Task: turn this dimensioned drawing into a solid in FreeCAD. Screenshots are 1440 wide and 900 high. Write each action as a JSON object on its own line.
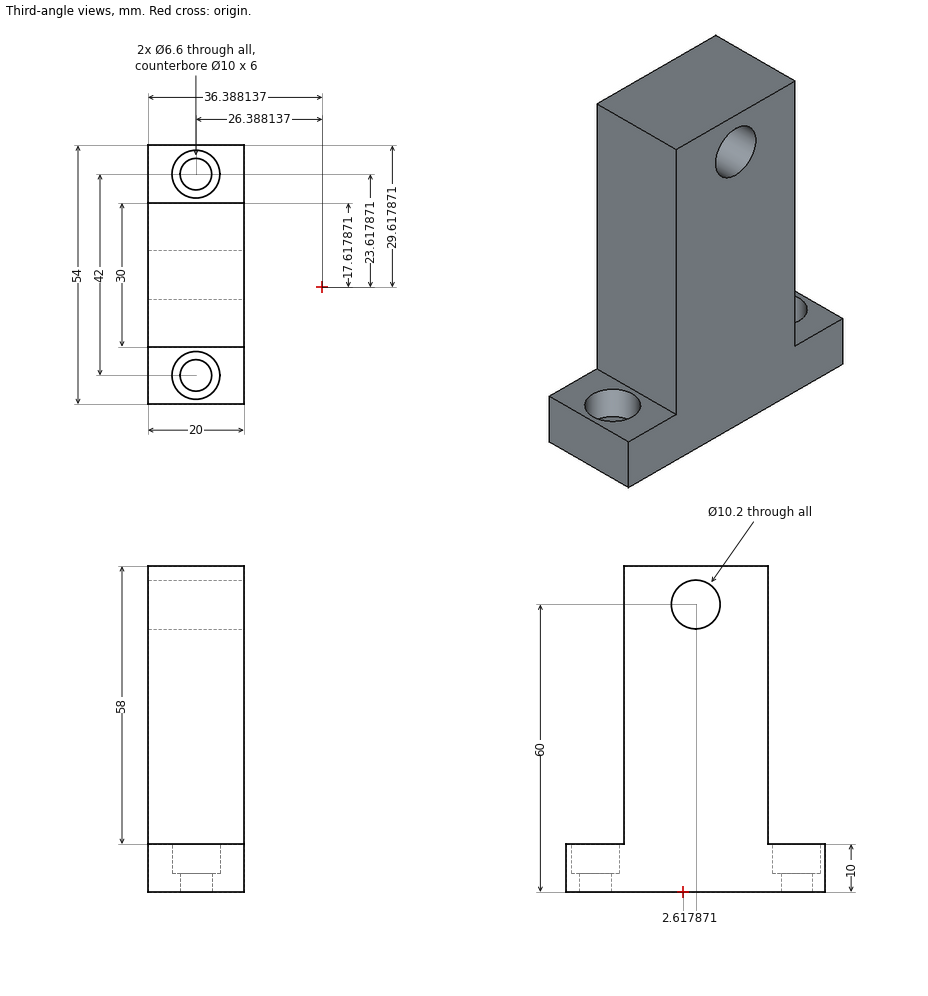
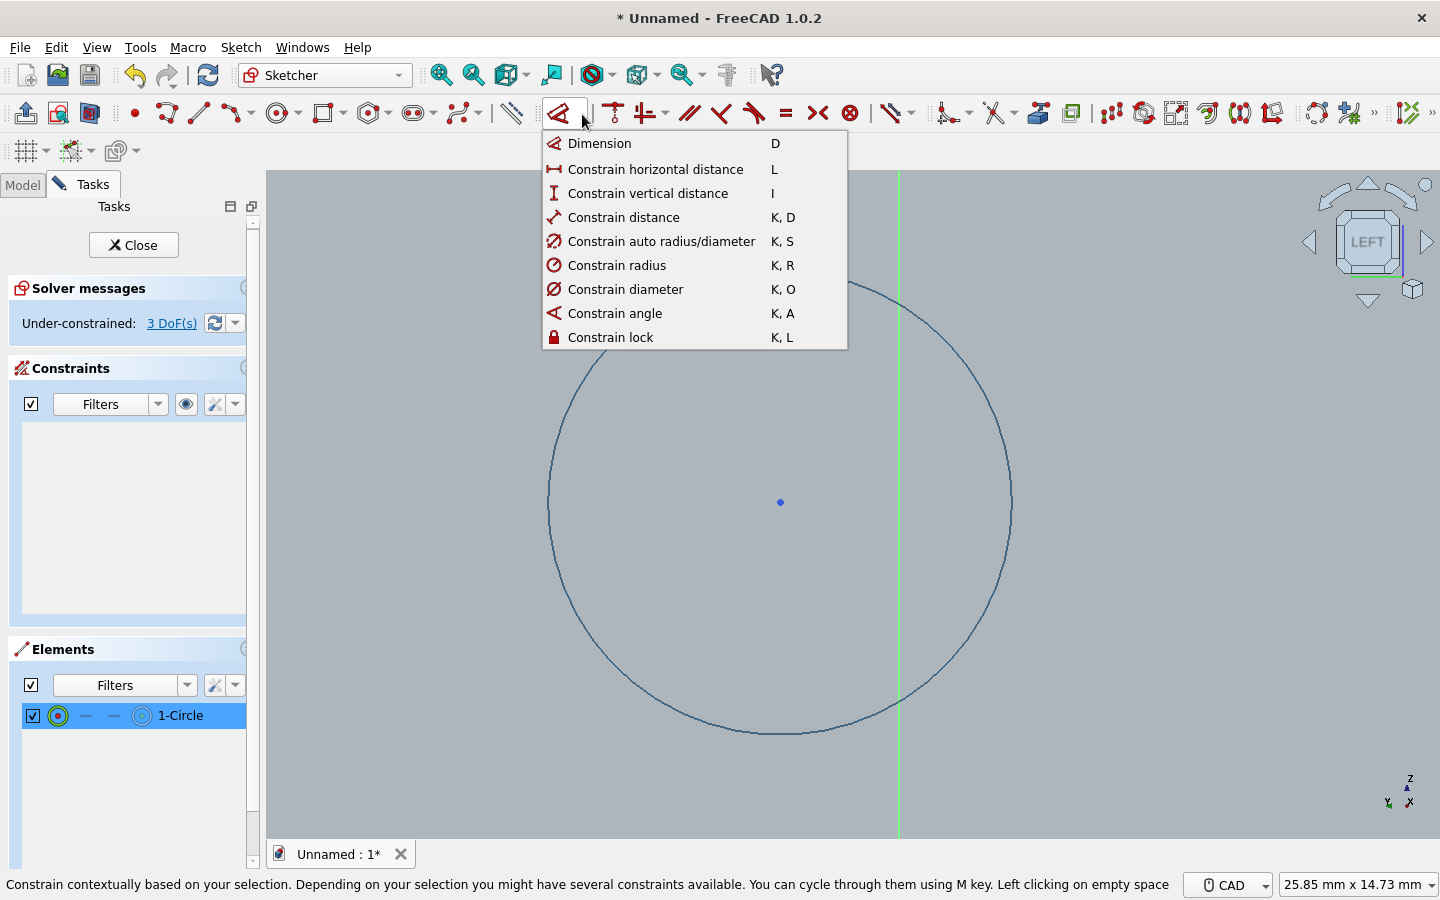
{"action": "left_click", "coordinate": [695, 289]}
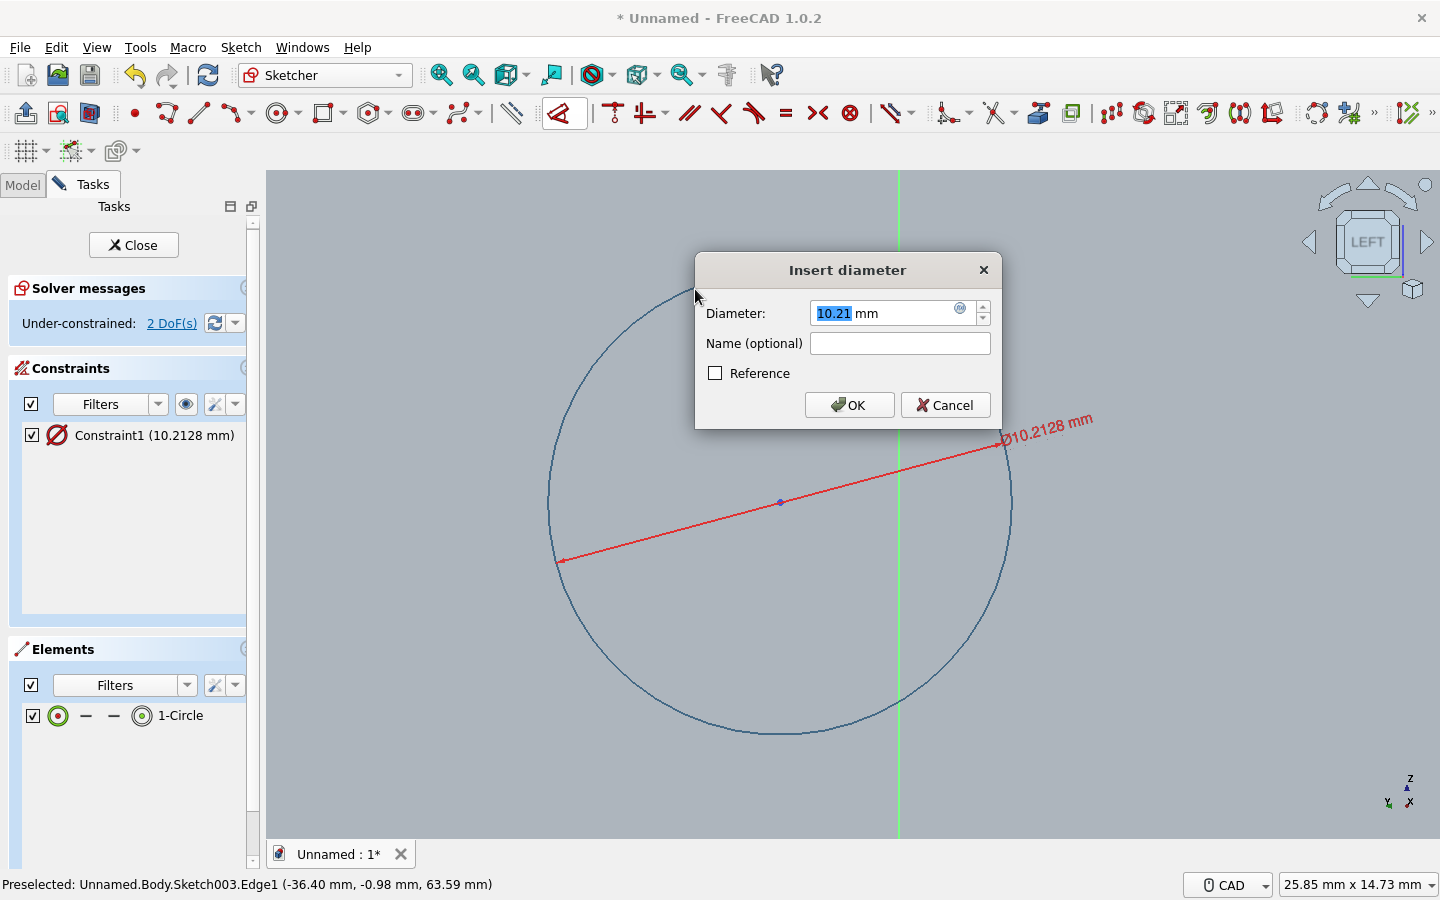
{"action": "type", "text": "10.2"}
{"action": "key", "text": "Return"}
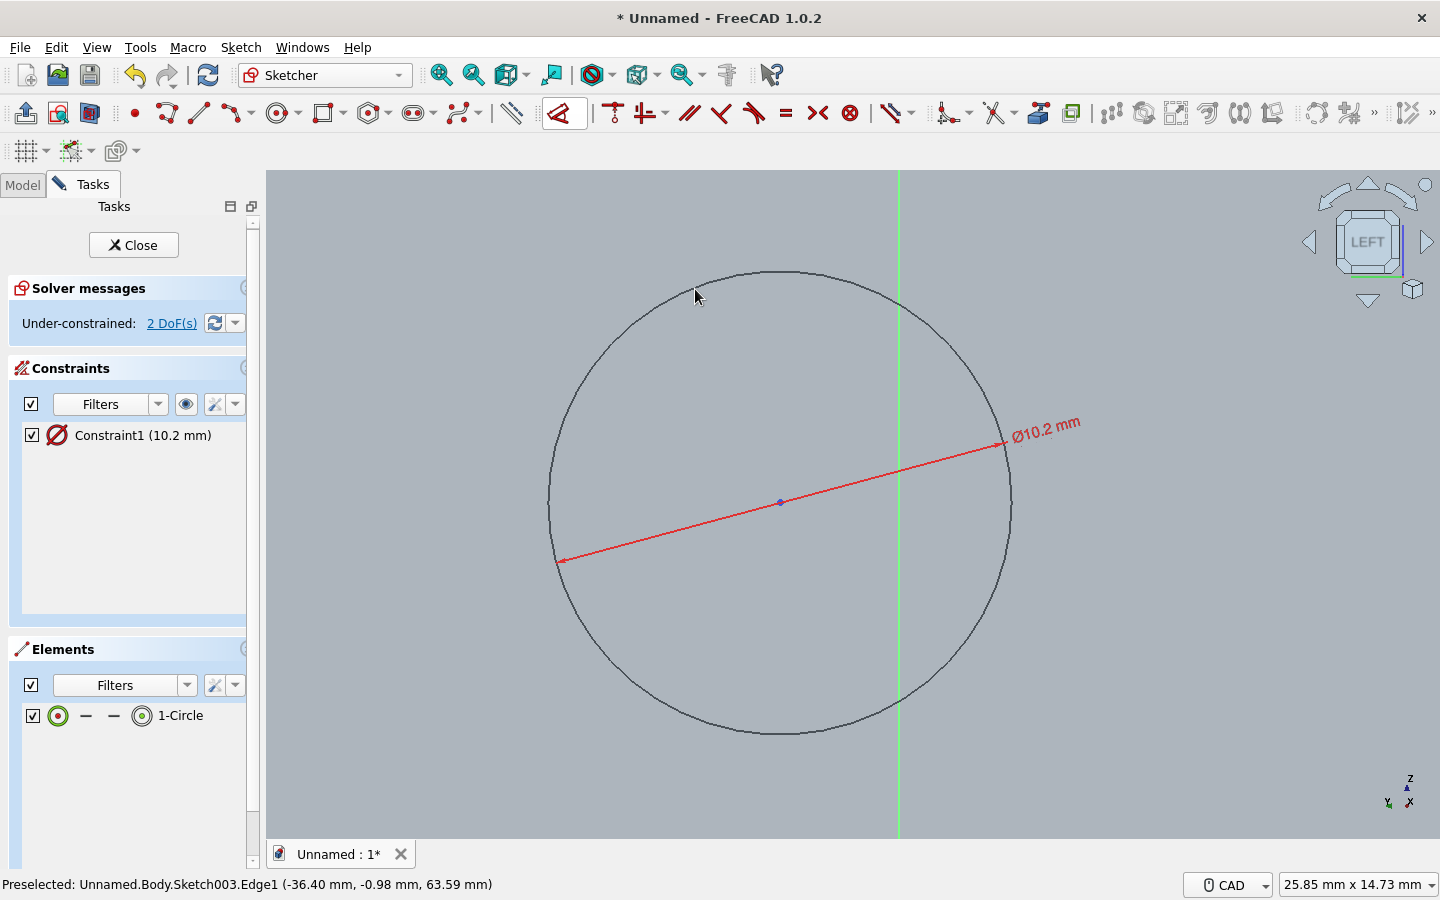
{"action": "left_click", "coordinate": [780, 503]}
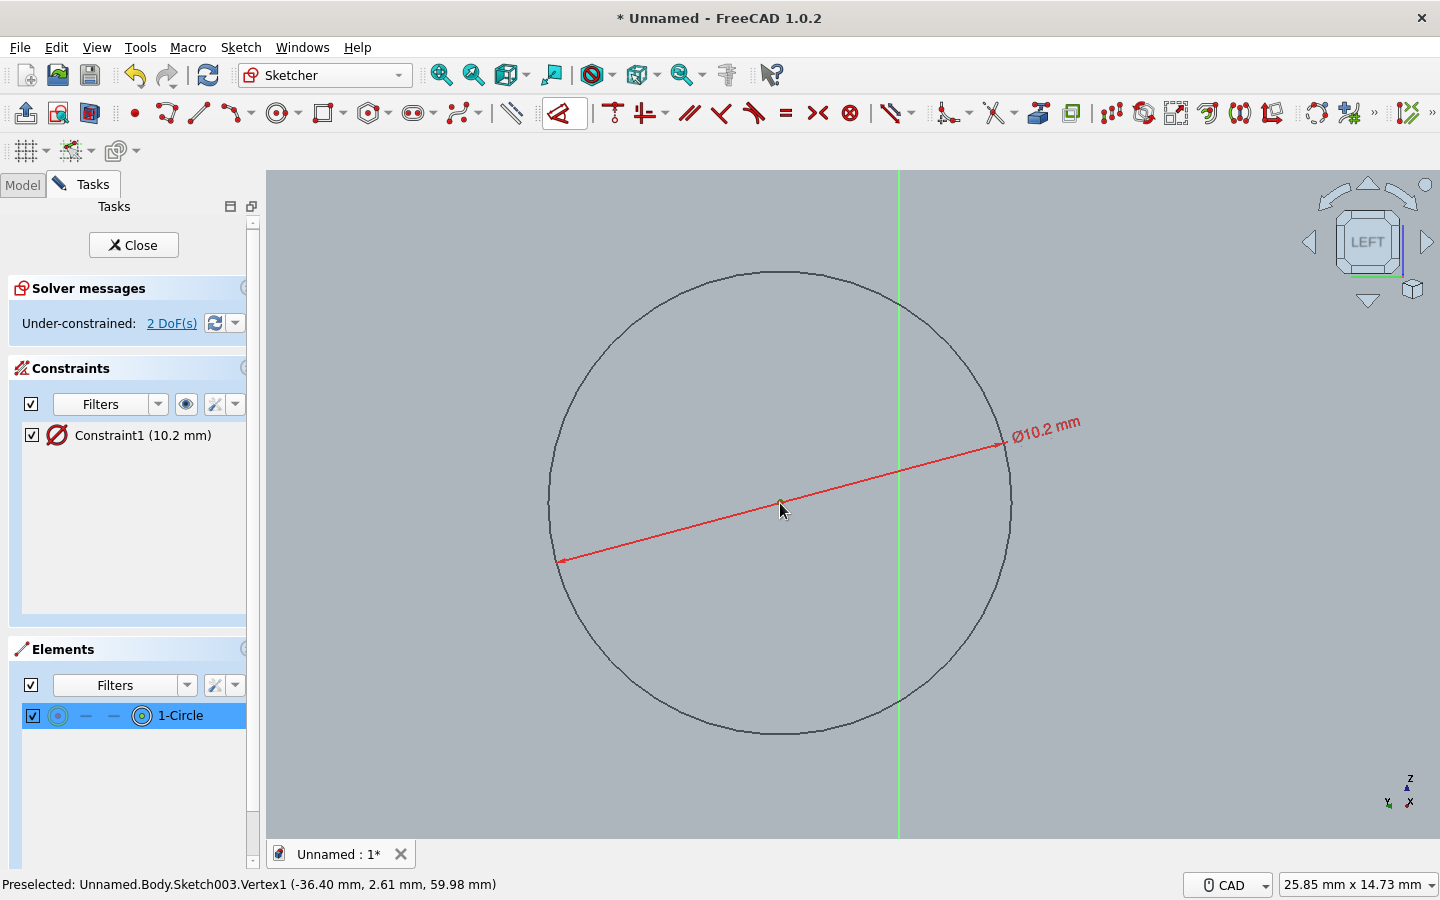
{"action": "key", "text": "i"}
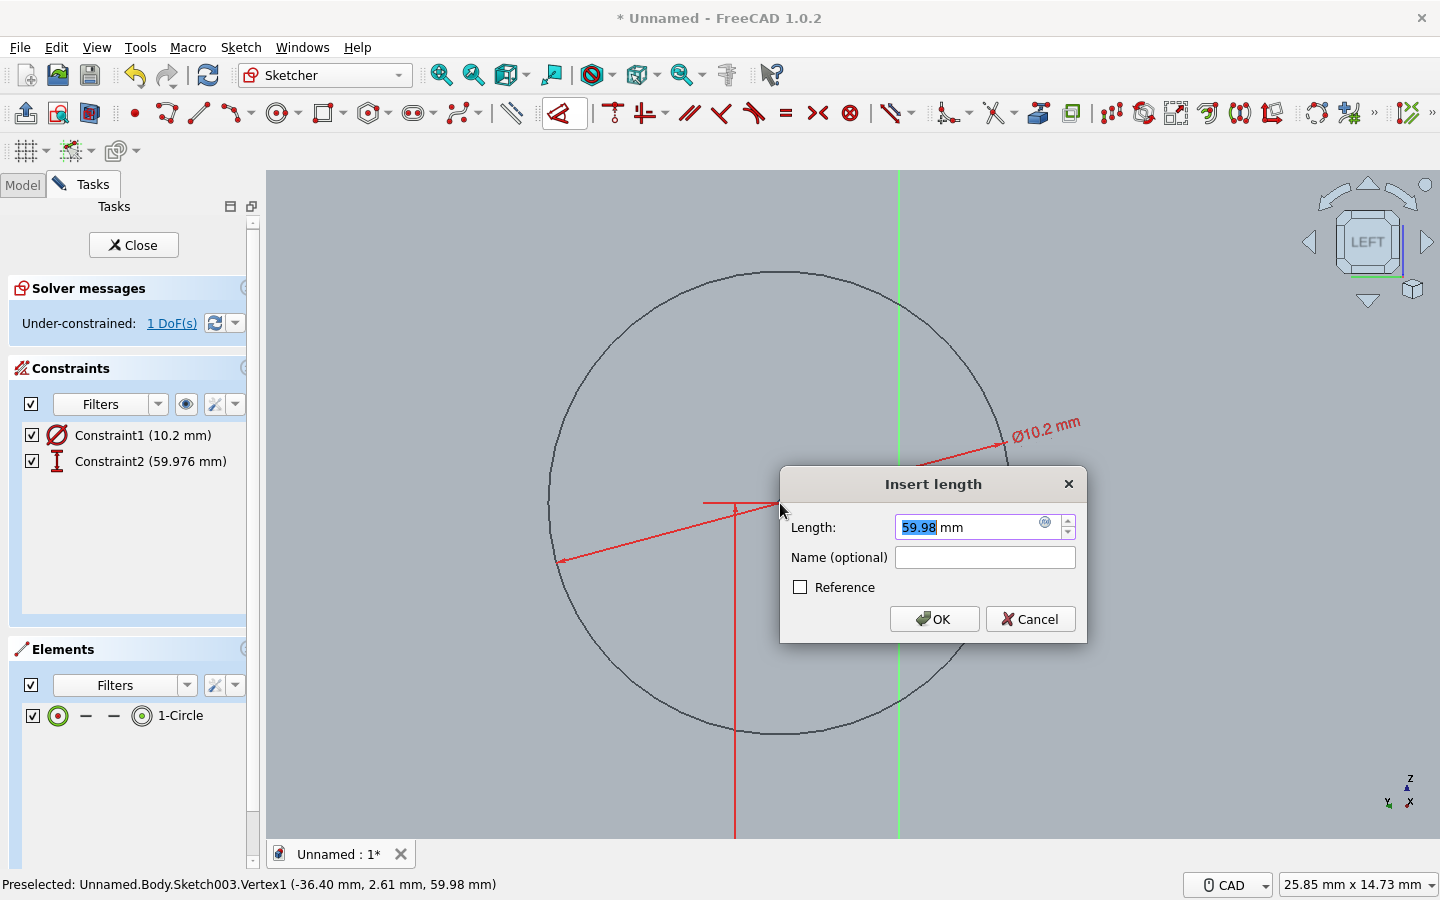
{"action": "type", "text": "60"}
{"action": "key", "text": "Return"}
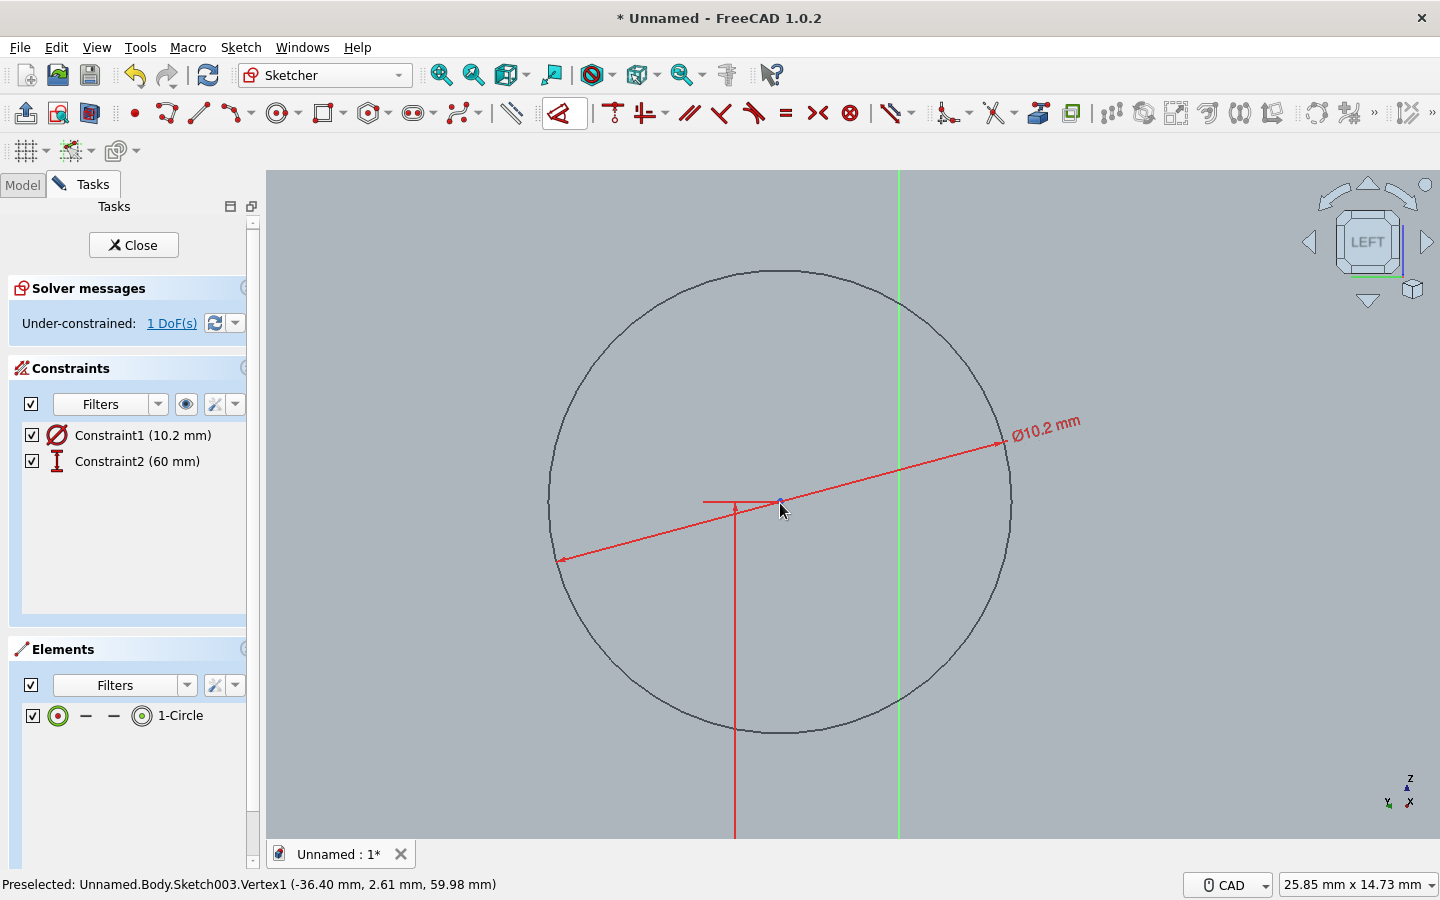
{"action": "left_click", "coordinate": [780, 502]}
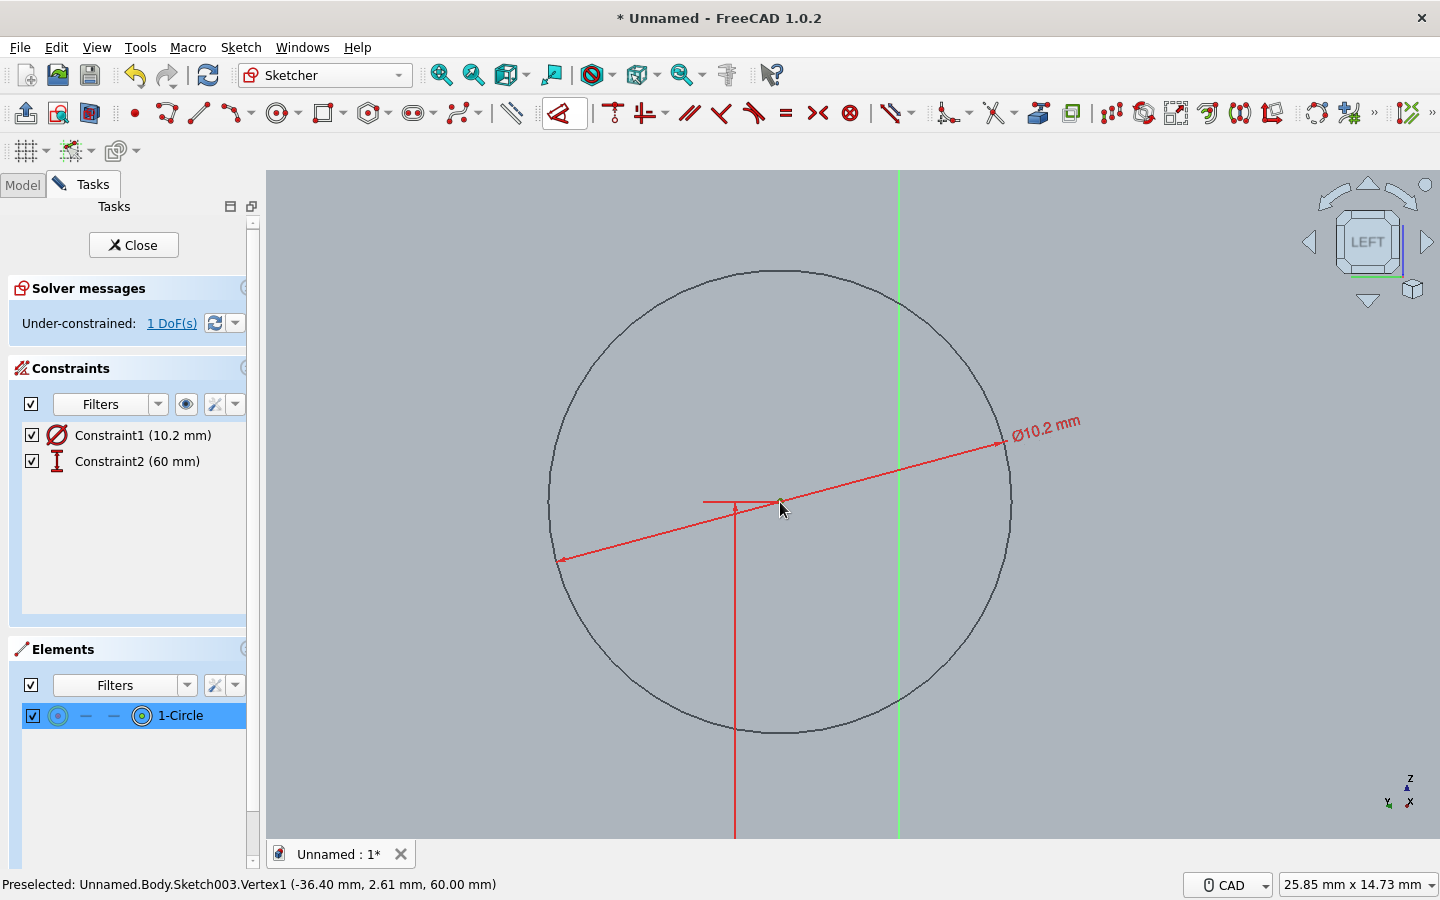
{"action": "key", "text": "l"}